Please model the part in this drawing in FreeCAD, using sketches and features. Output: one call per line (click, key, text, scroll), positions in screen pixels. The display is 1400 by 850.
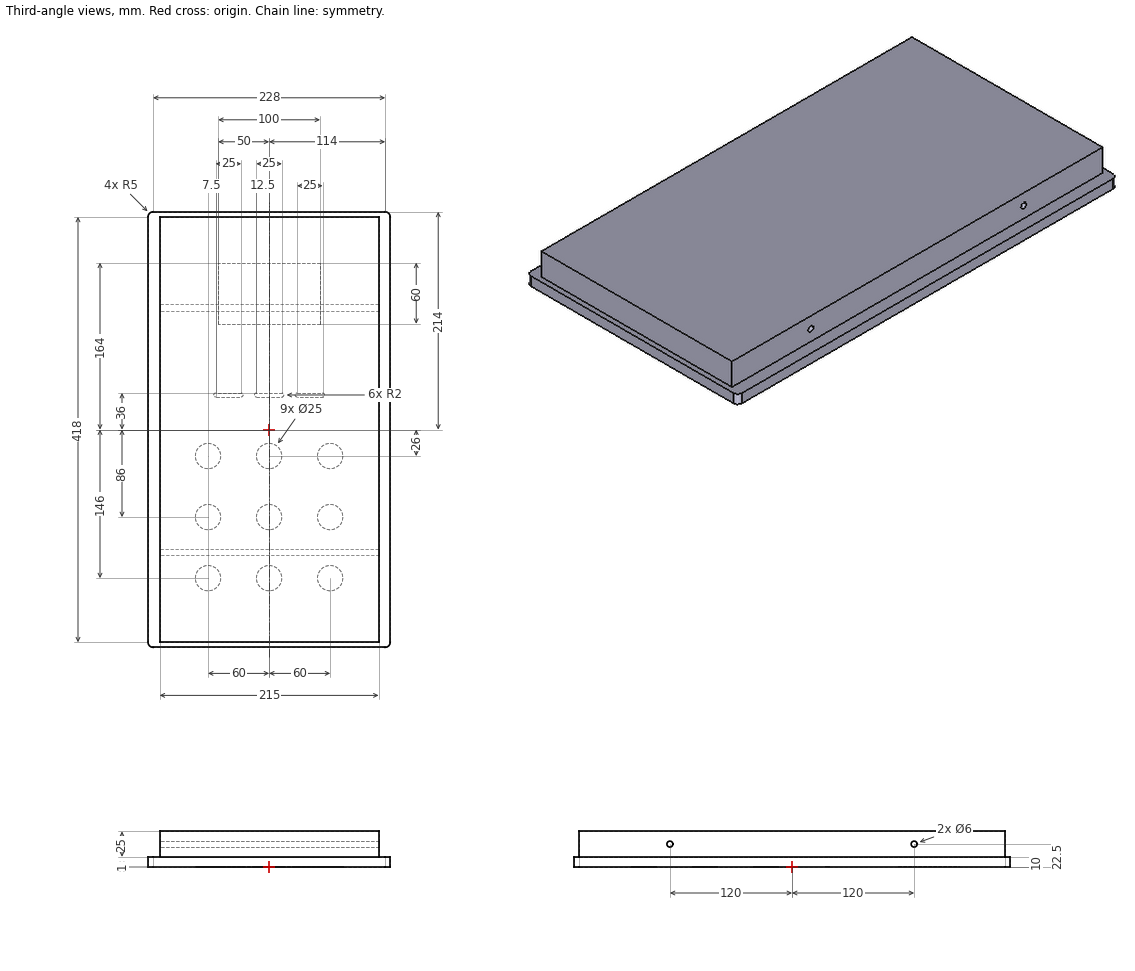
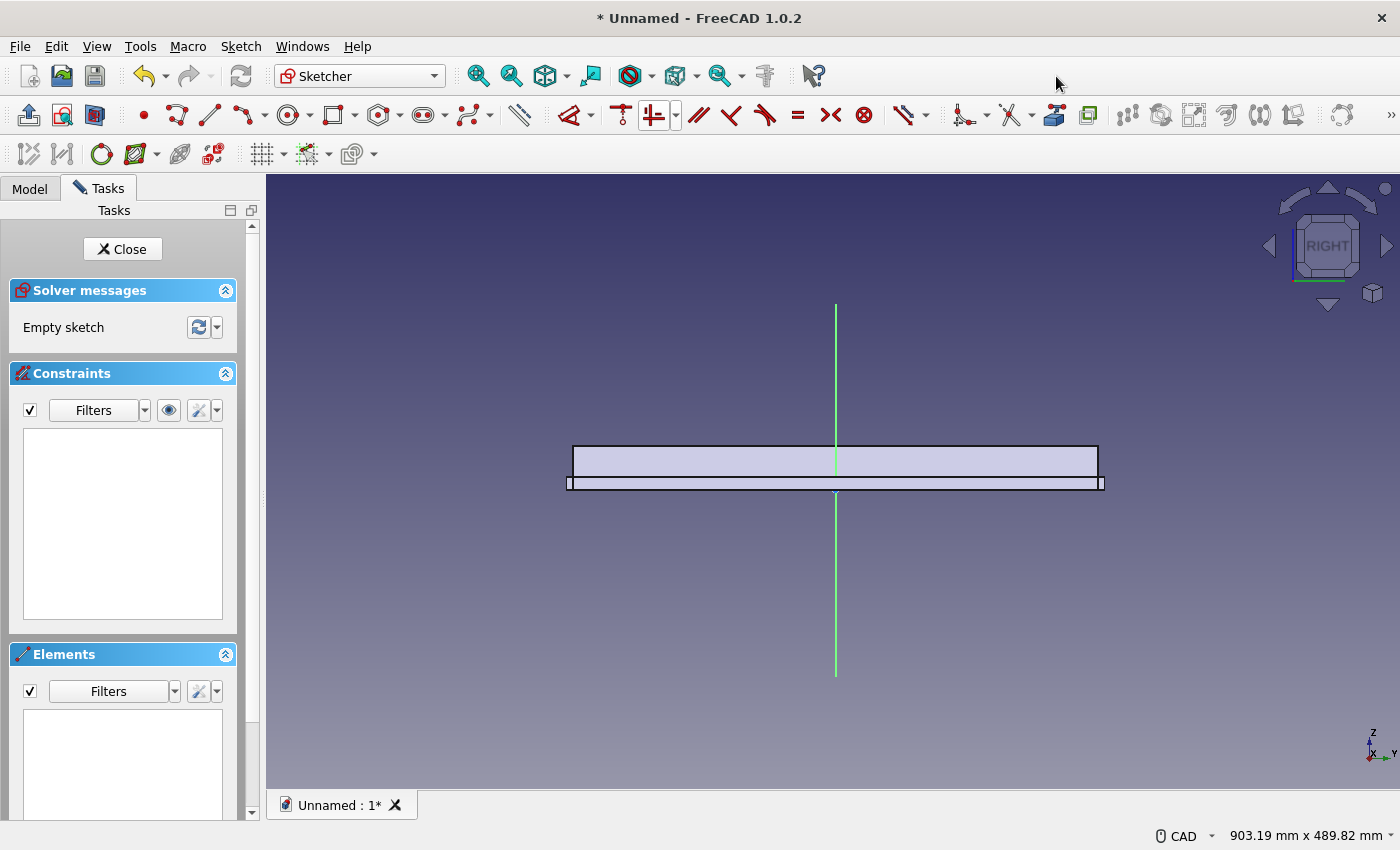
click(95, 116)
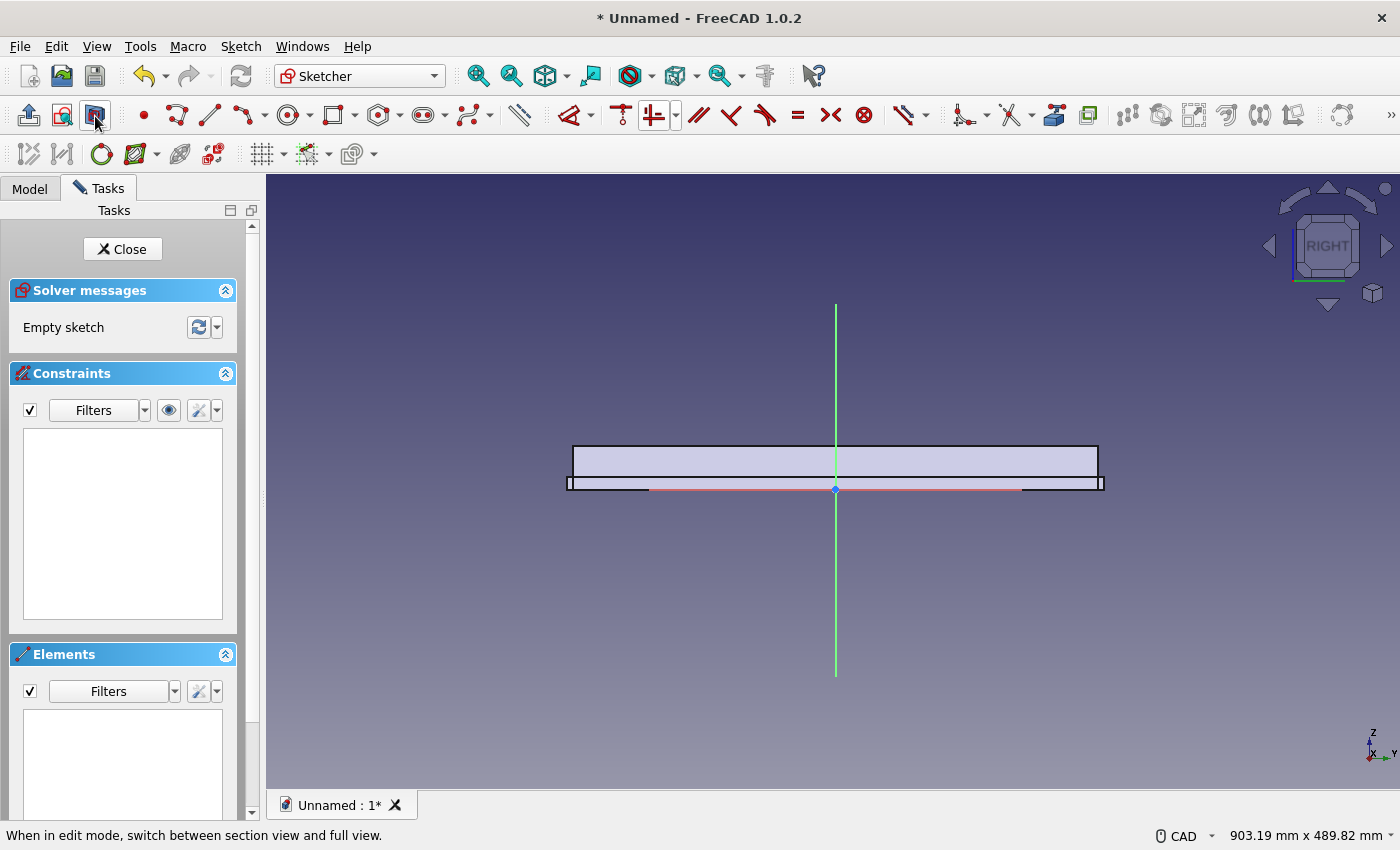
scroll(894, 467, up, 4)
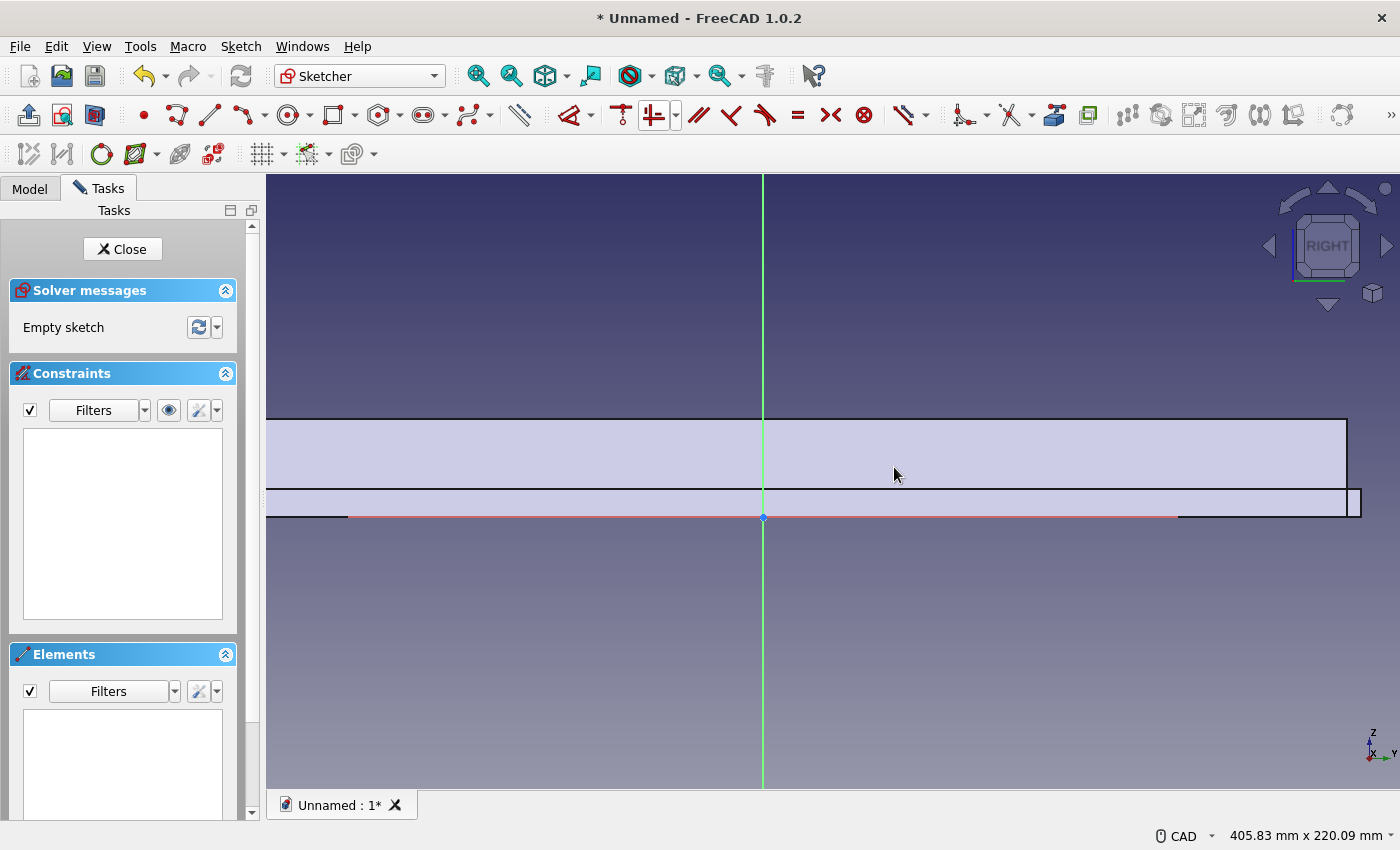
click(288, 116)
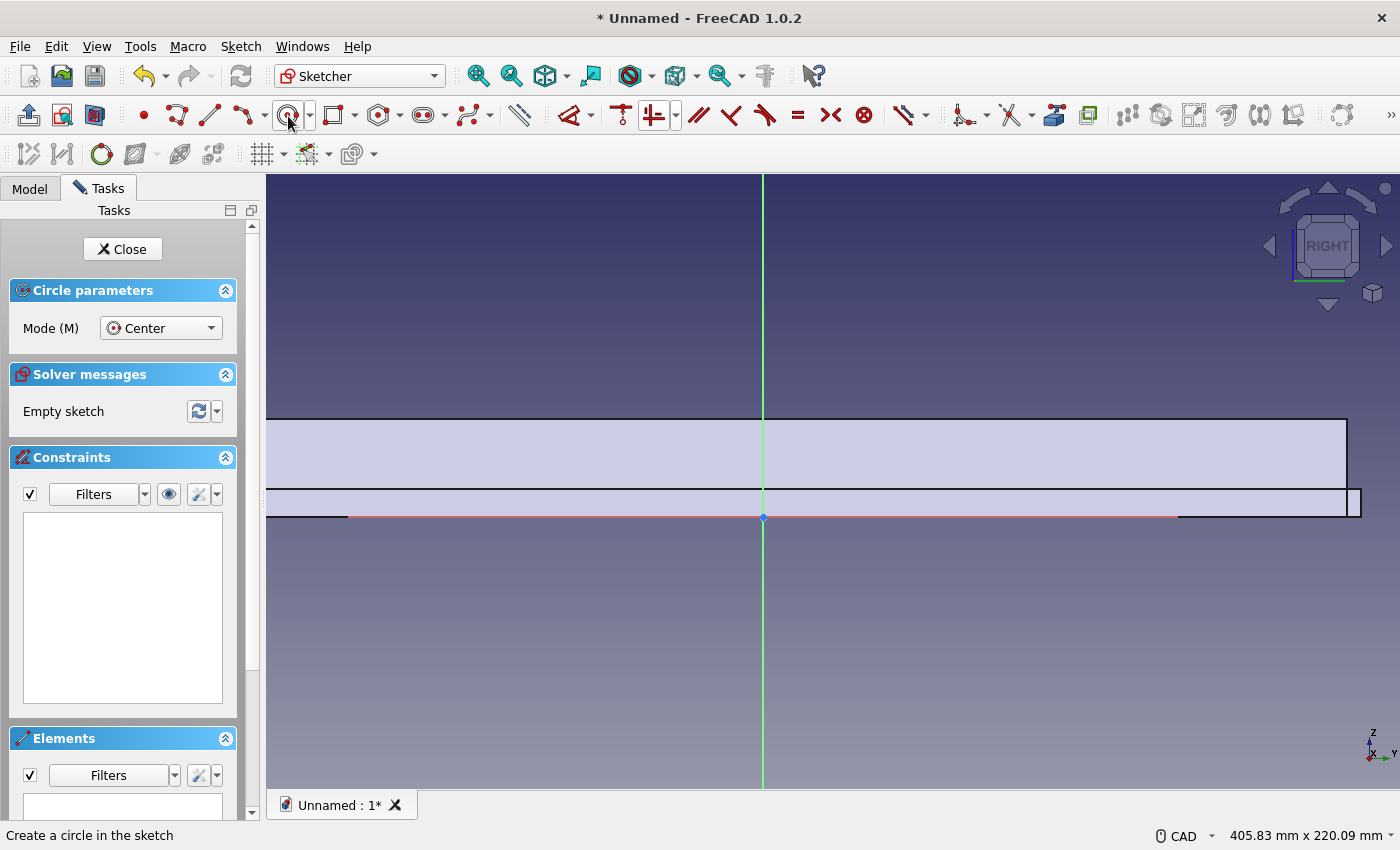
scroll(1099, 454, up, 5)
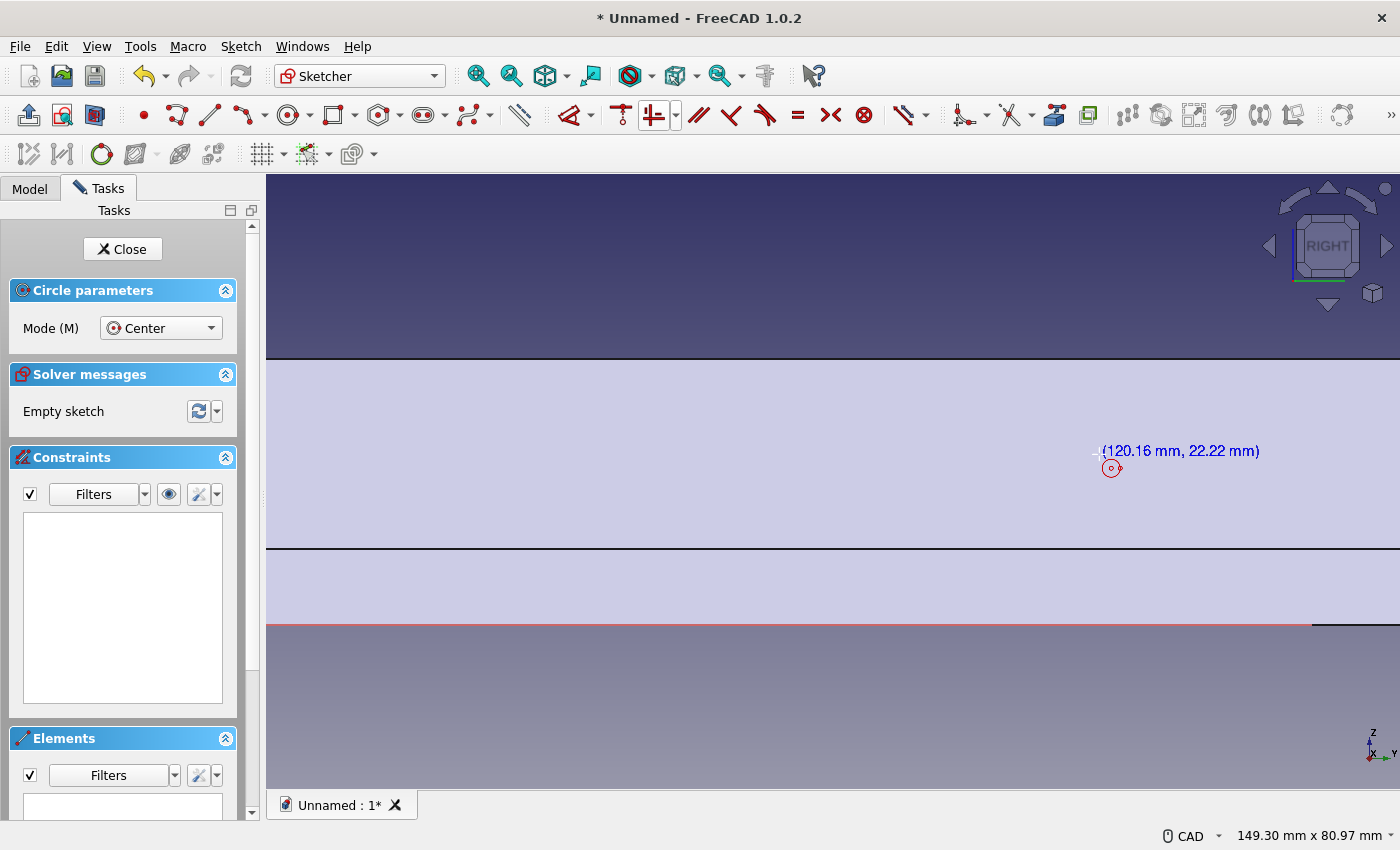
click(1097, 454)
move(1113, 438)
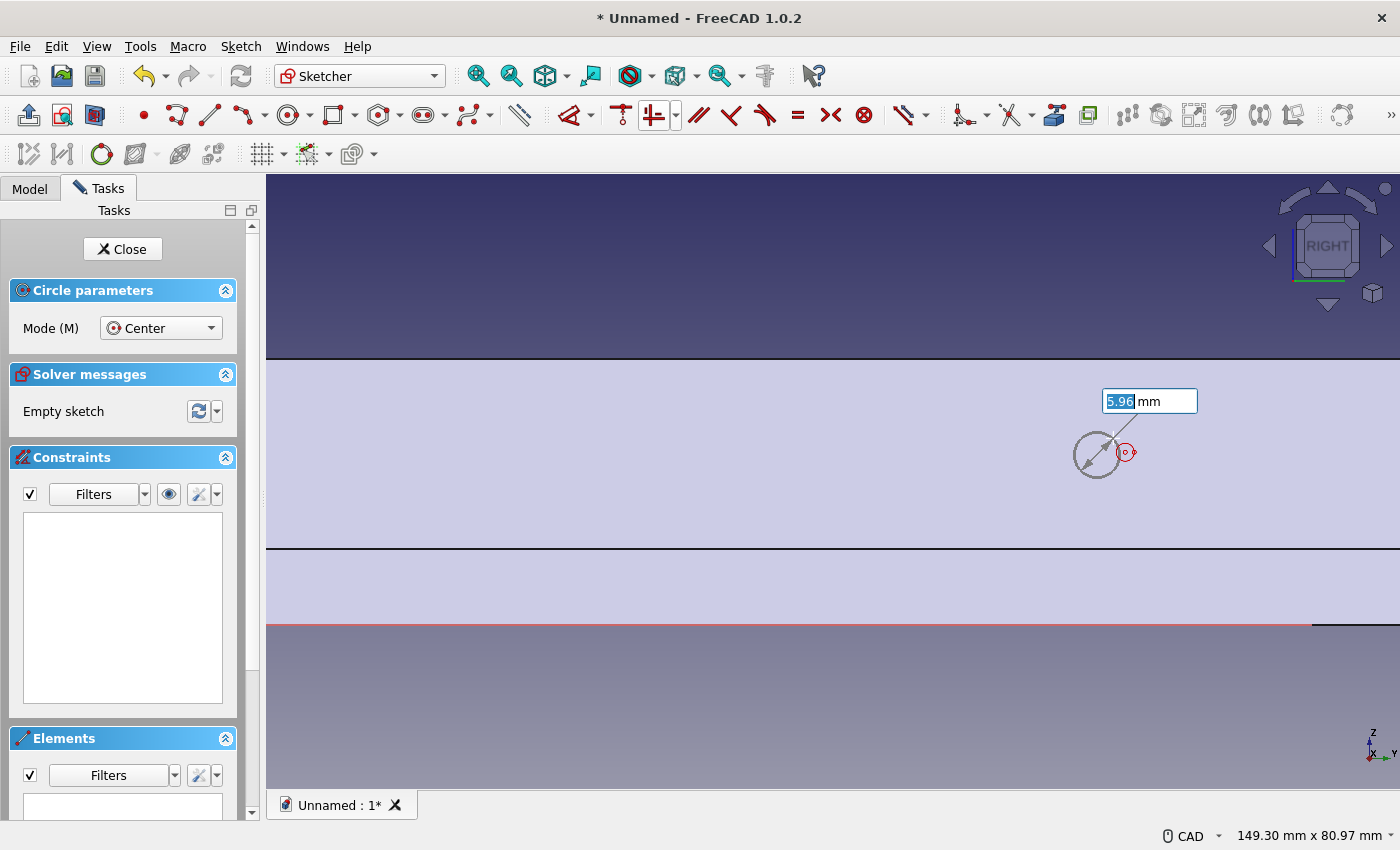
text(6)
key(Return)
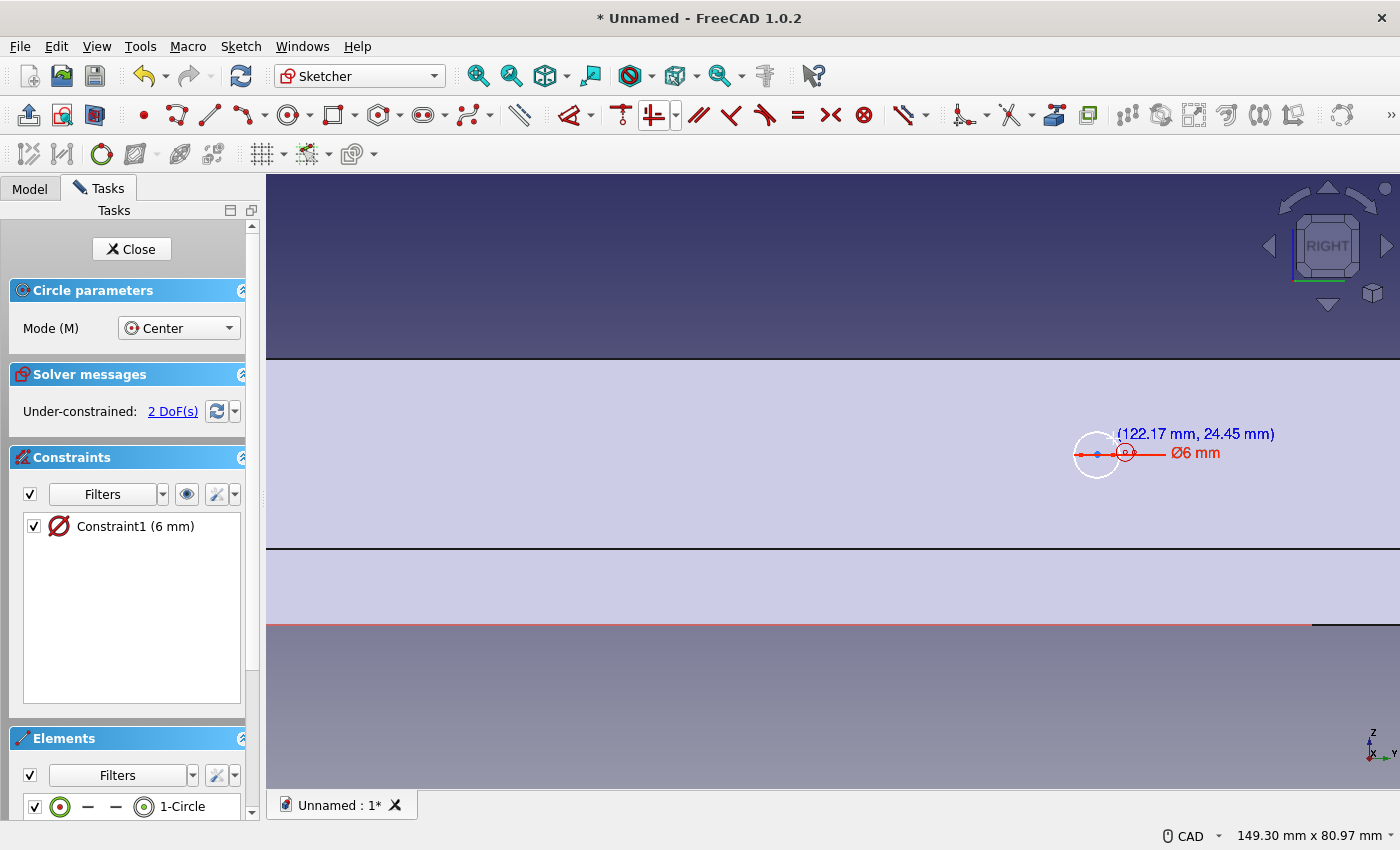
scroll(1102, 455, down, 5)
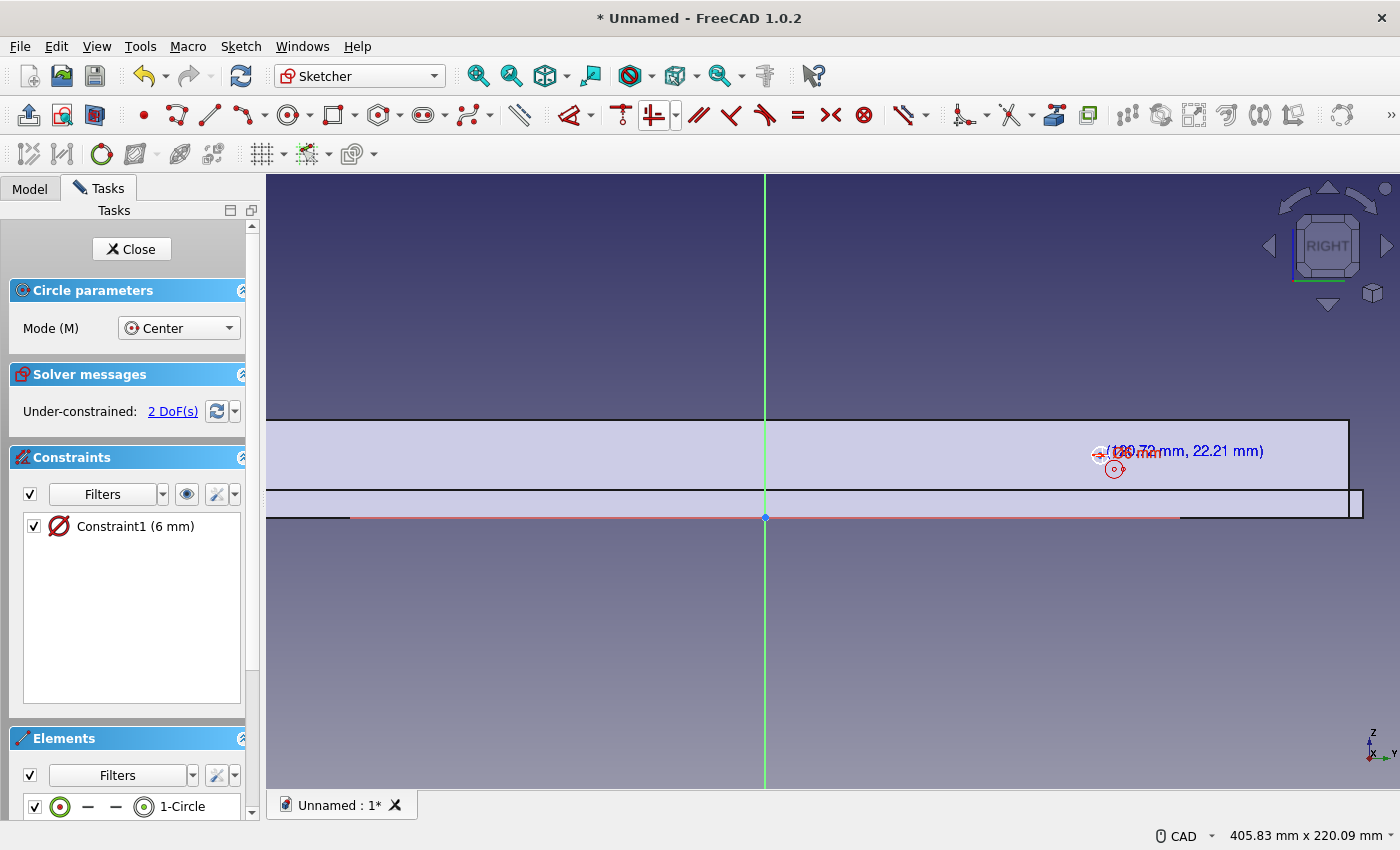
scroll(430, 455, up, 5)